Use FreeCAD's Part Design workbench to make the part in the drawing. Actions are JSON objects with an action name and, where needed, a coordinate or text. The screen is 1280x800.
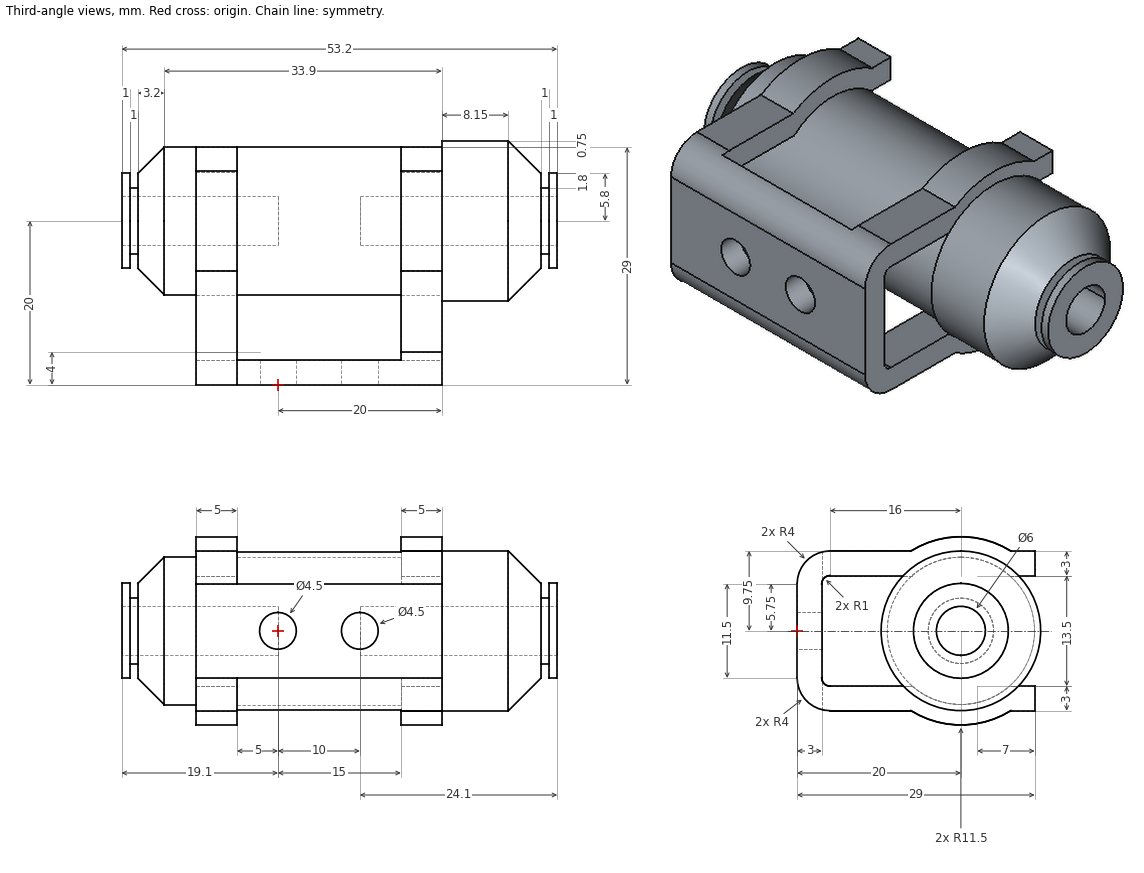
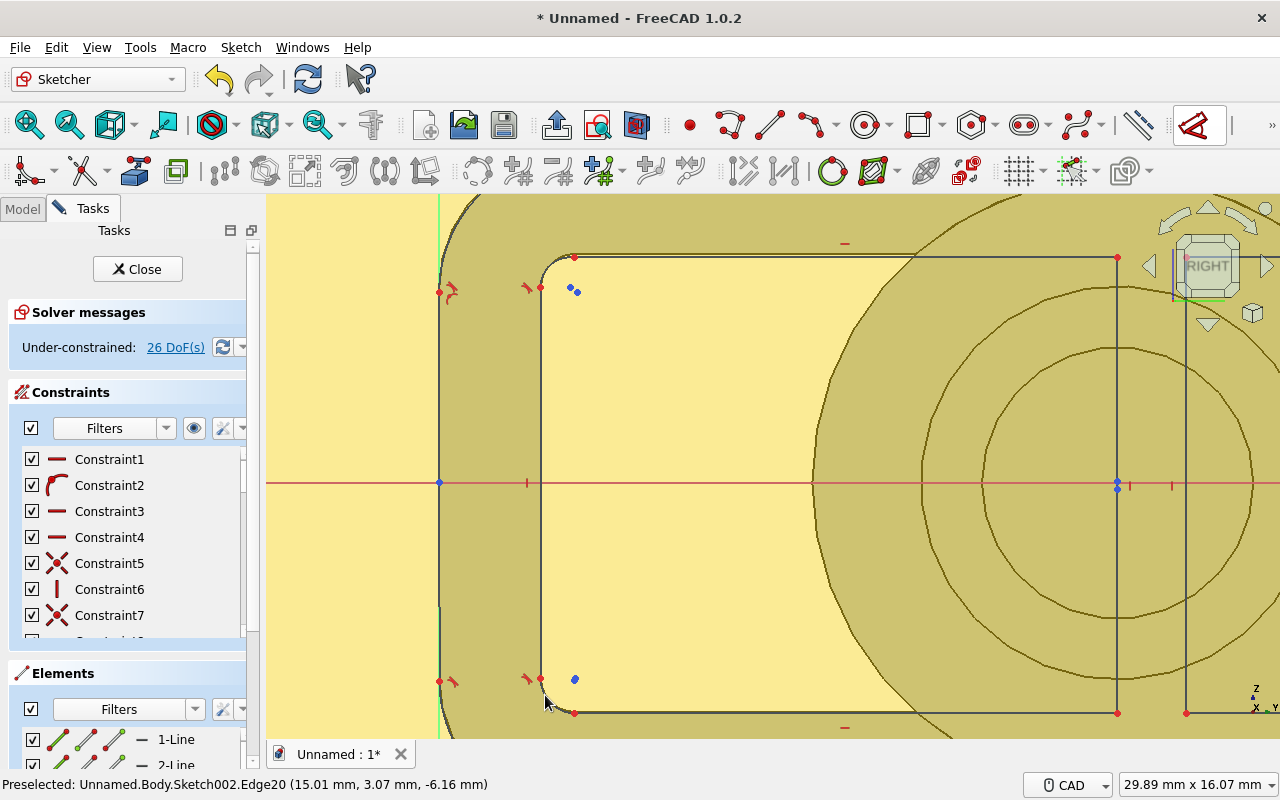
{"action": "left_click", "coordinate": [737, 257]}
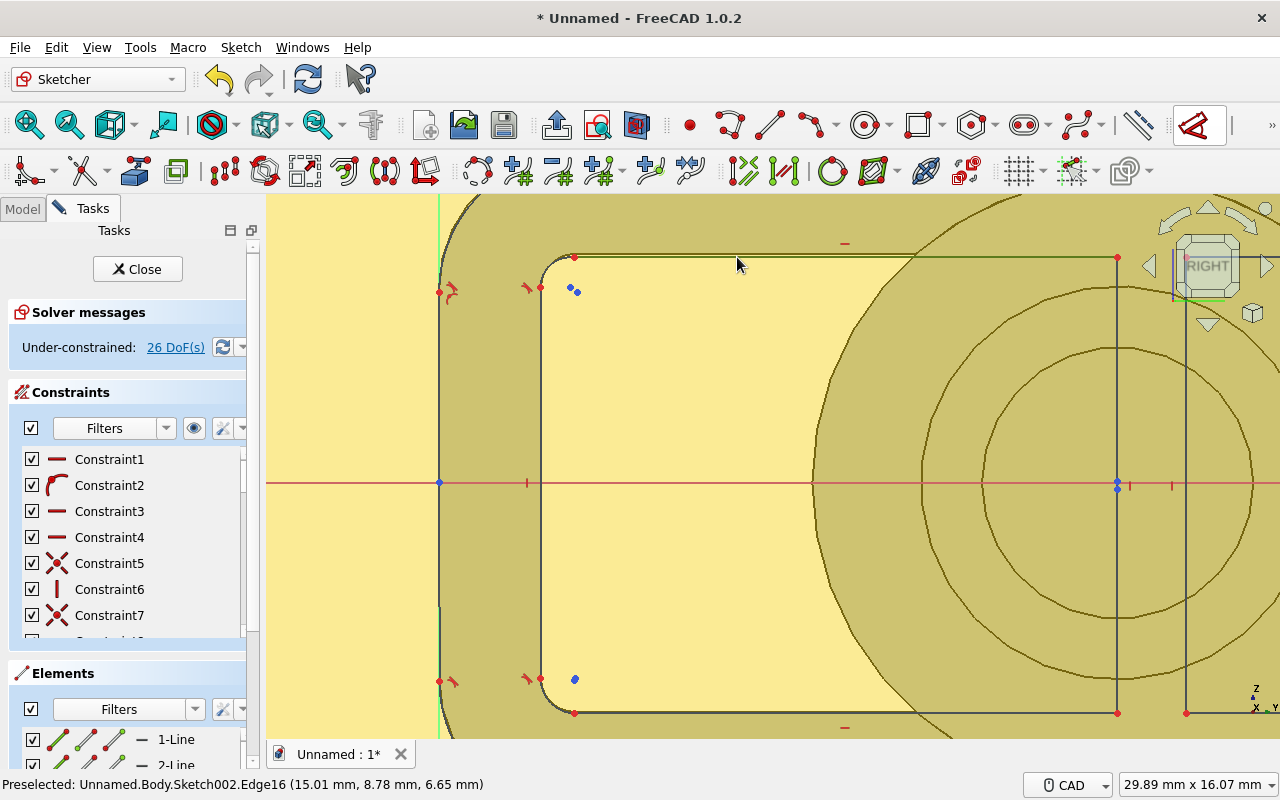
{"action": "left_click", "coordinate": [559, 259]}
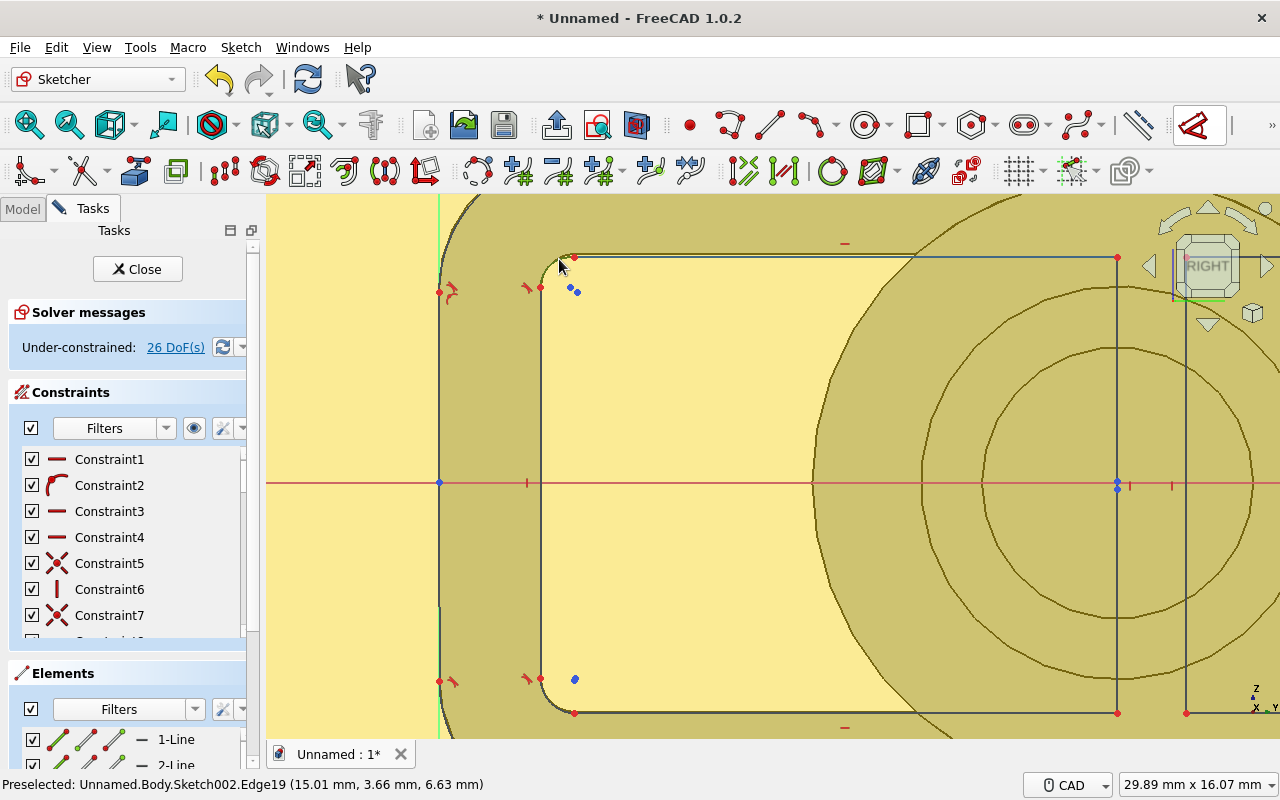
{"action": "key", "text": "t"}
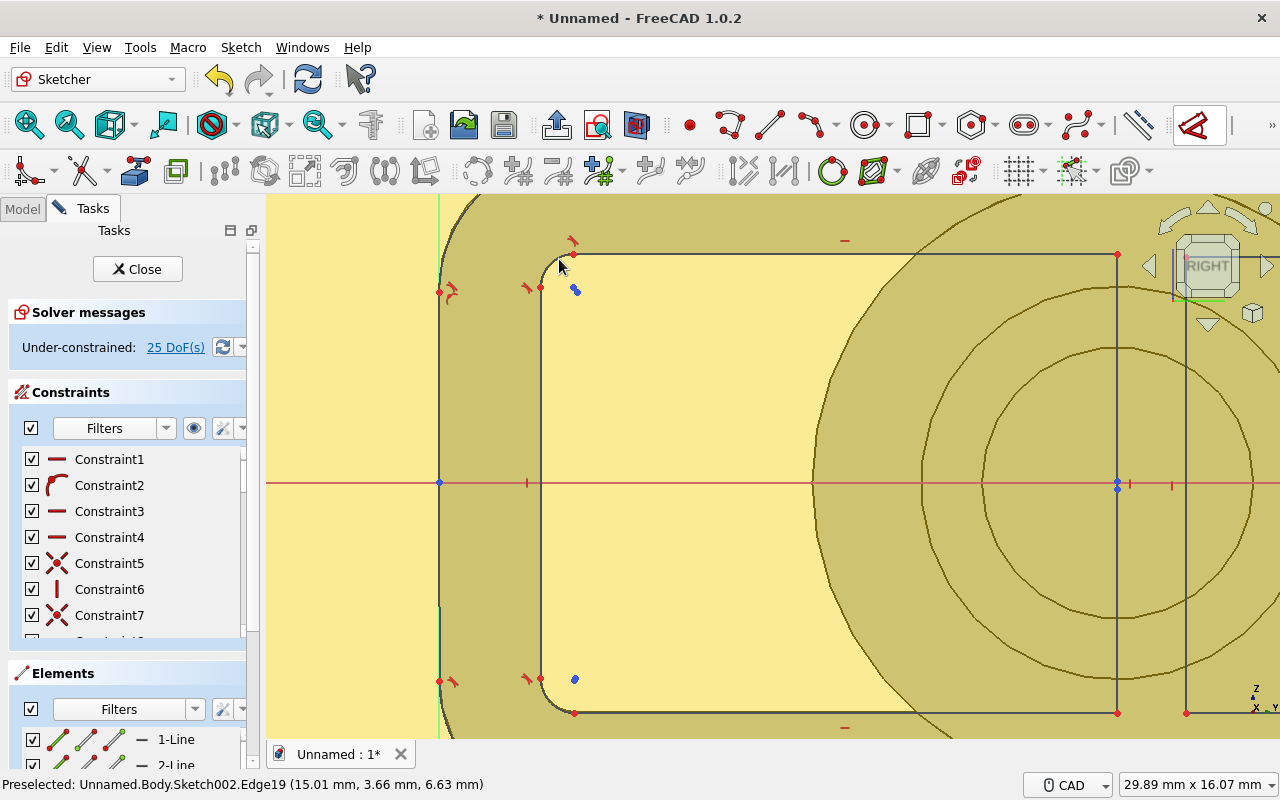
{"action": "scroll", "coordinate": [520, 453], "scroll_direction": "down", "scroll_amount": 4}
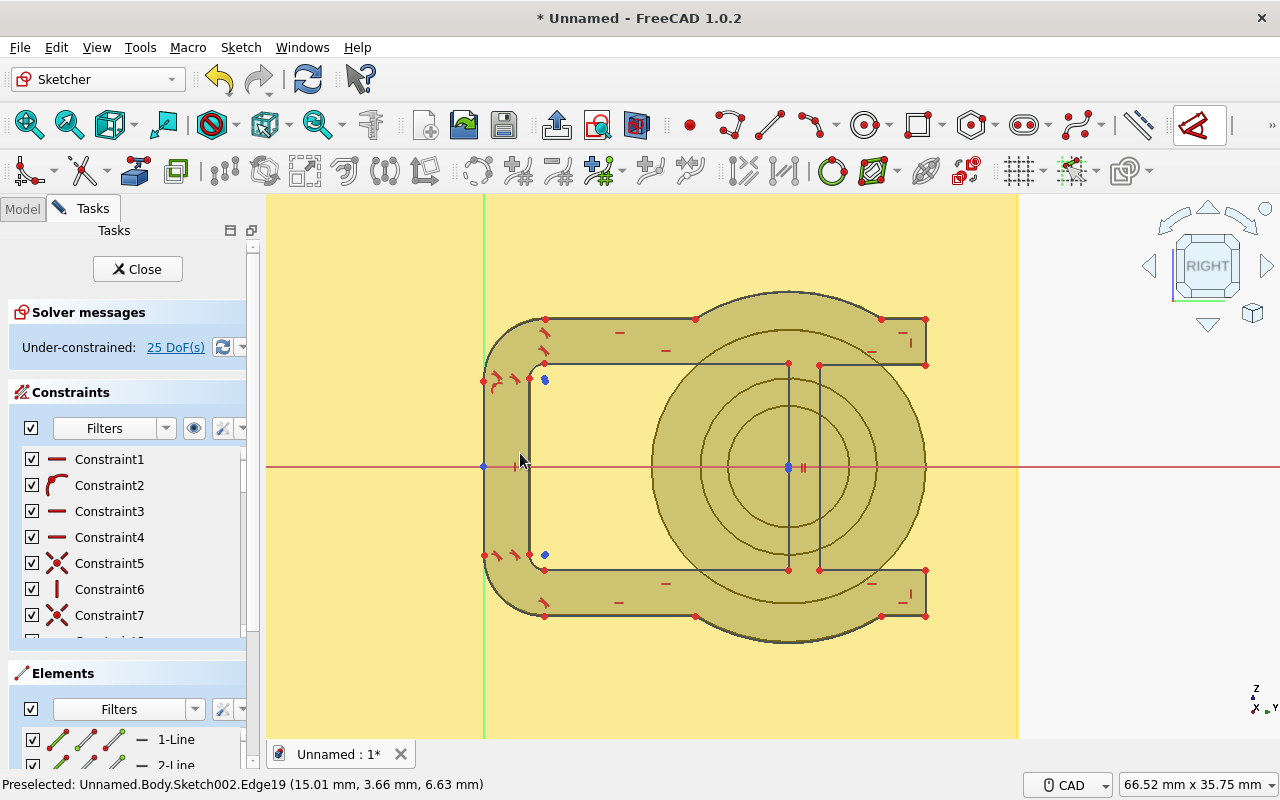
{"action": "left_click", "coordinate": [715, 570]}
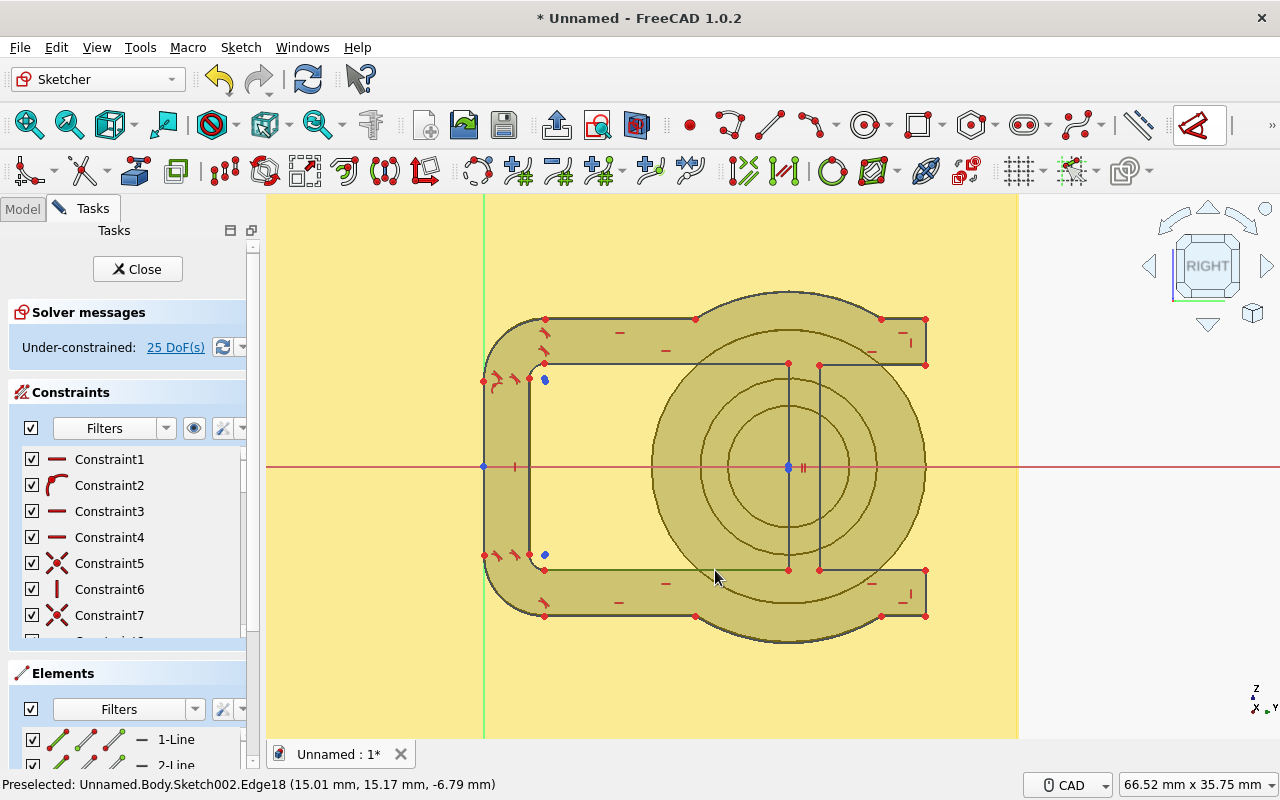
{"action": "left_click", "coordinate": [534, 565]}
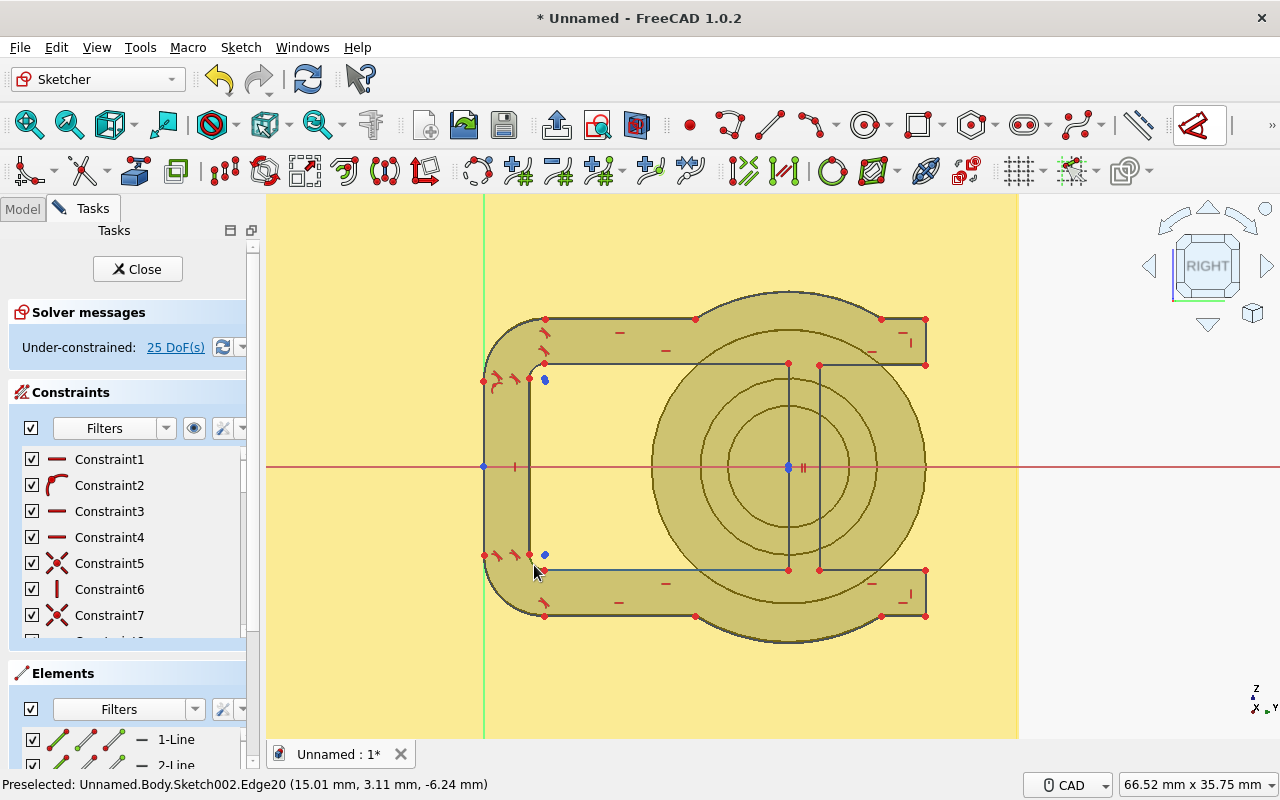
{"action": "key", "text": "t"}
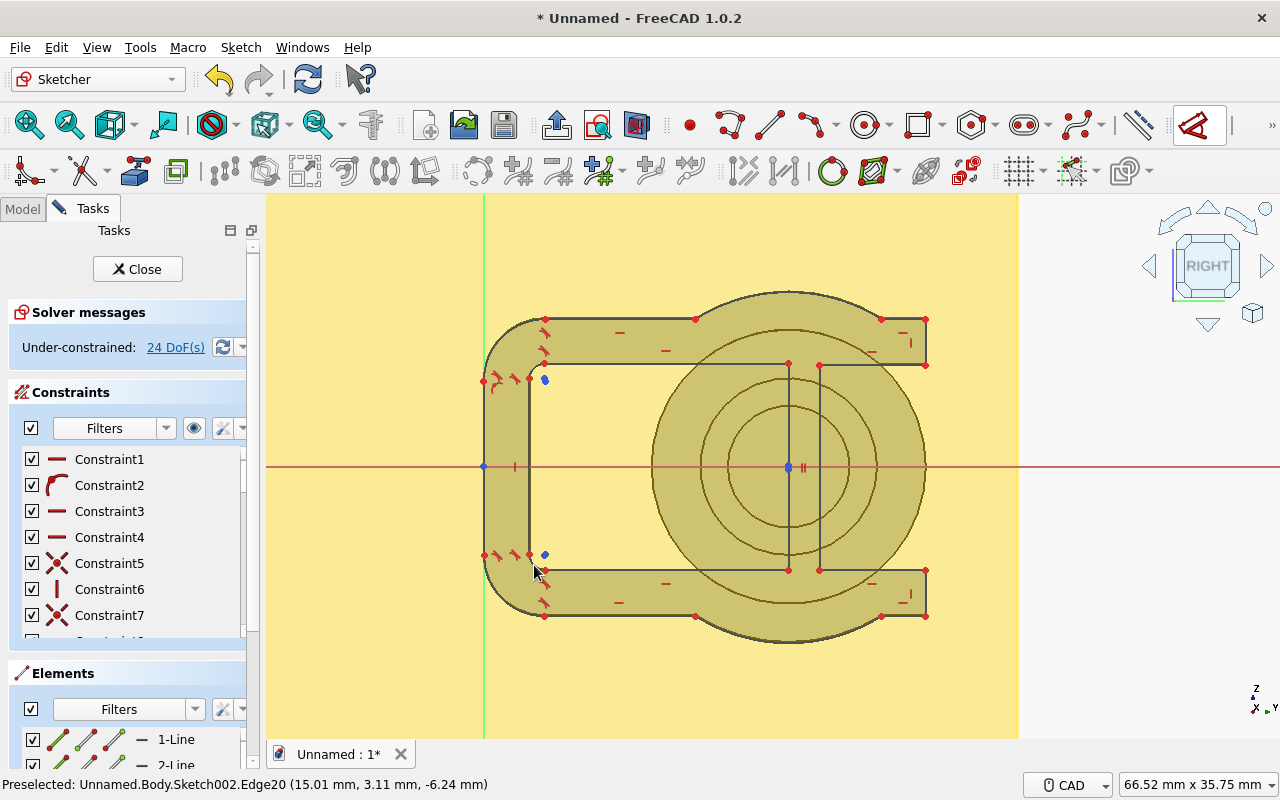
{"action": "left_click", "coordinate": [484, 434]}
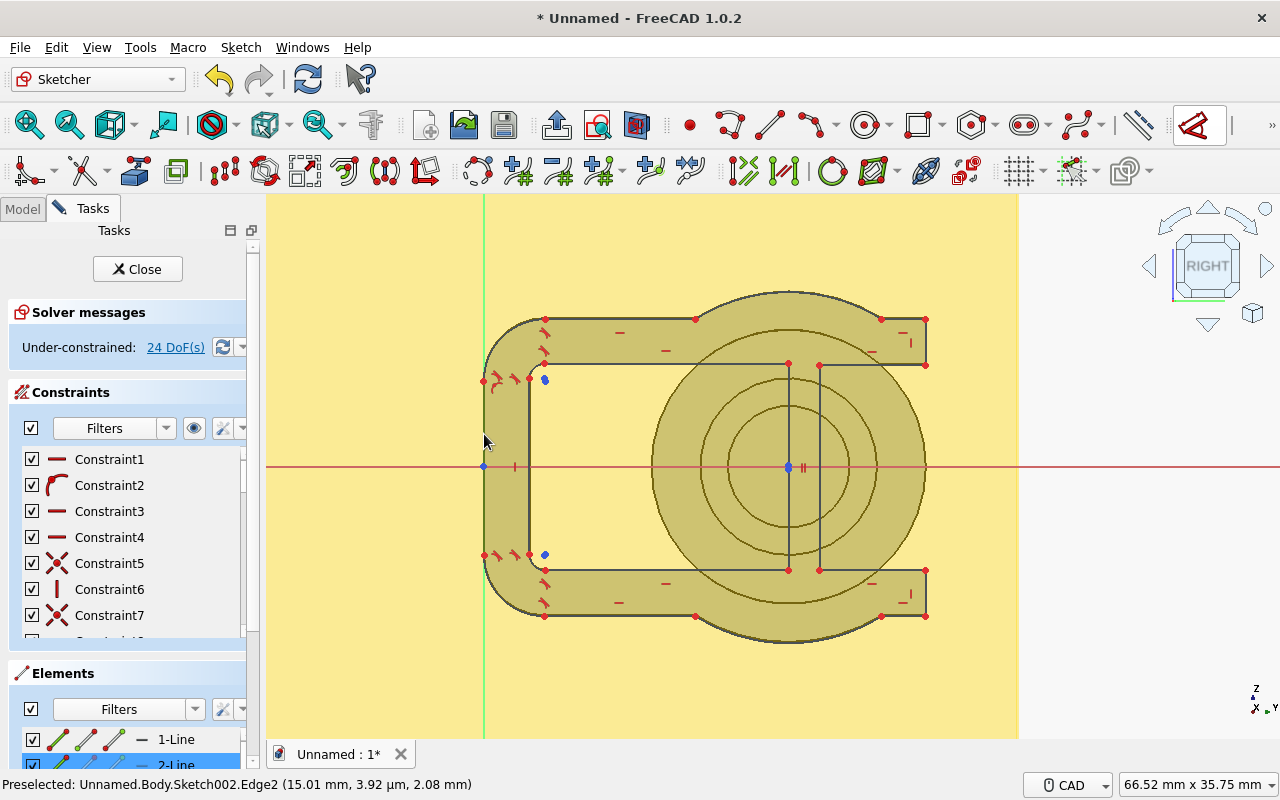
{"action": "key", "text": "v"}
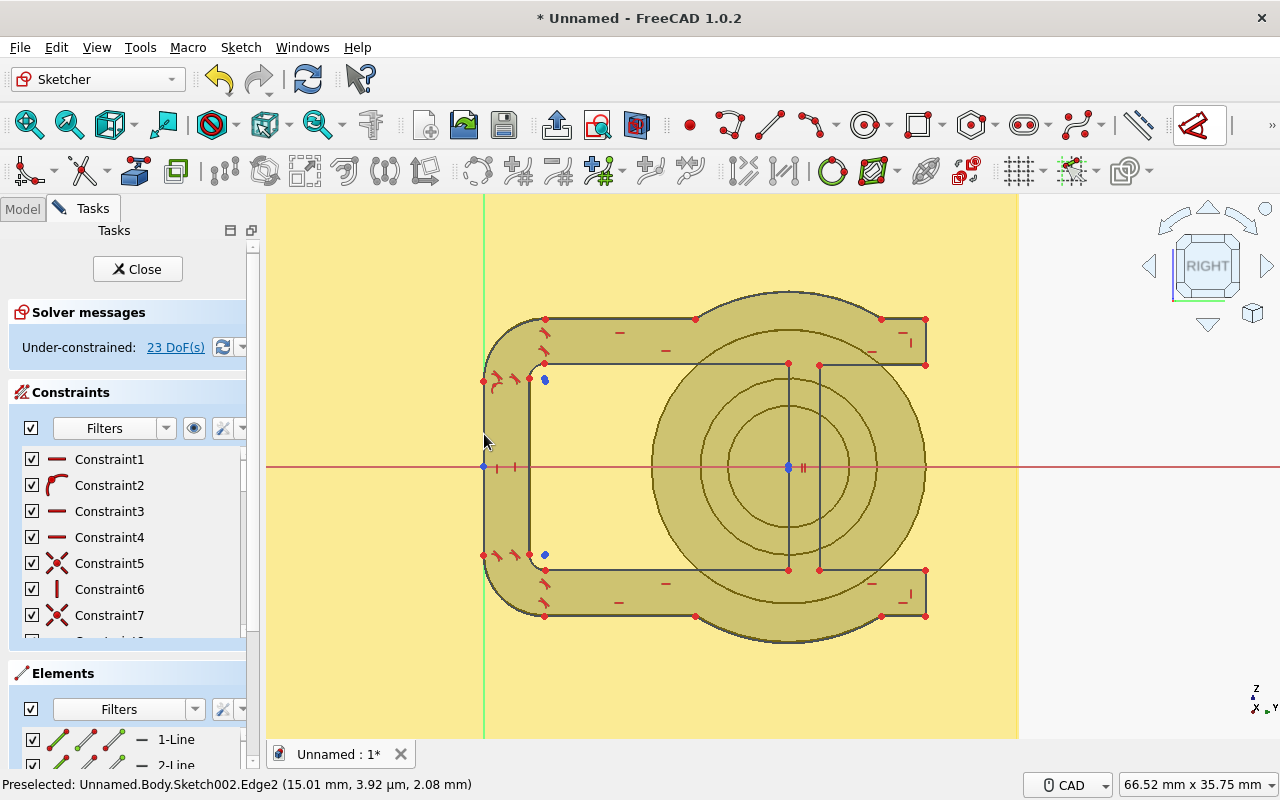
{"action": "left_click", "coordinate": [750, 639]}